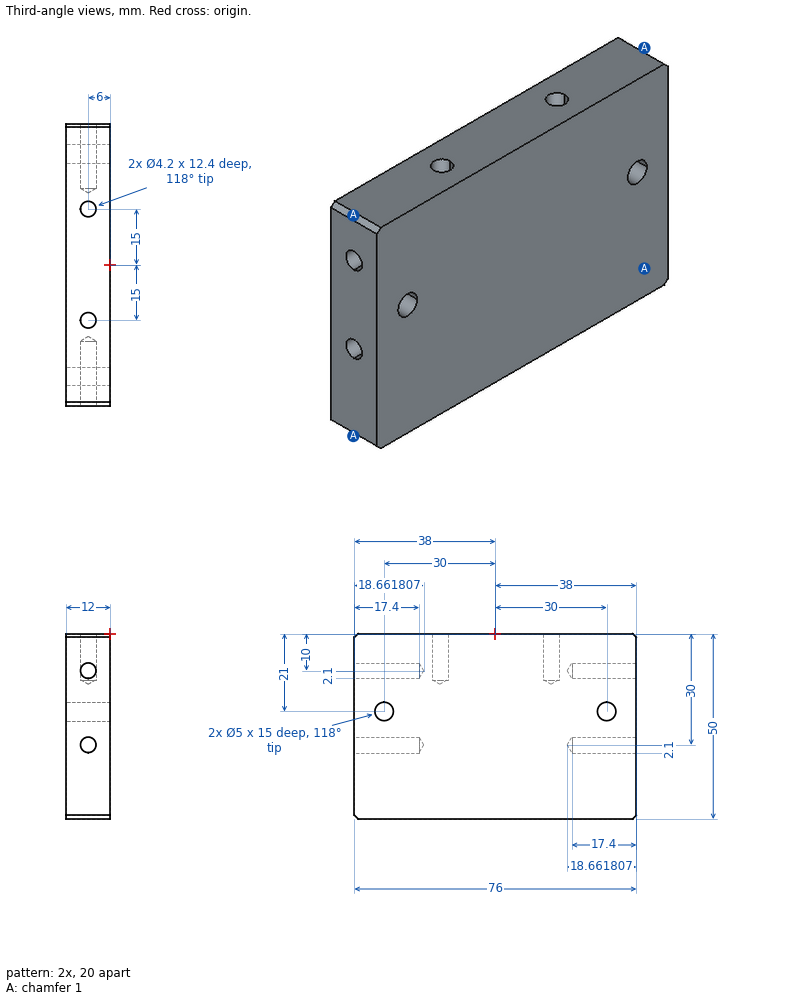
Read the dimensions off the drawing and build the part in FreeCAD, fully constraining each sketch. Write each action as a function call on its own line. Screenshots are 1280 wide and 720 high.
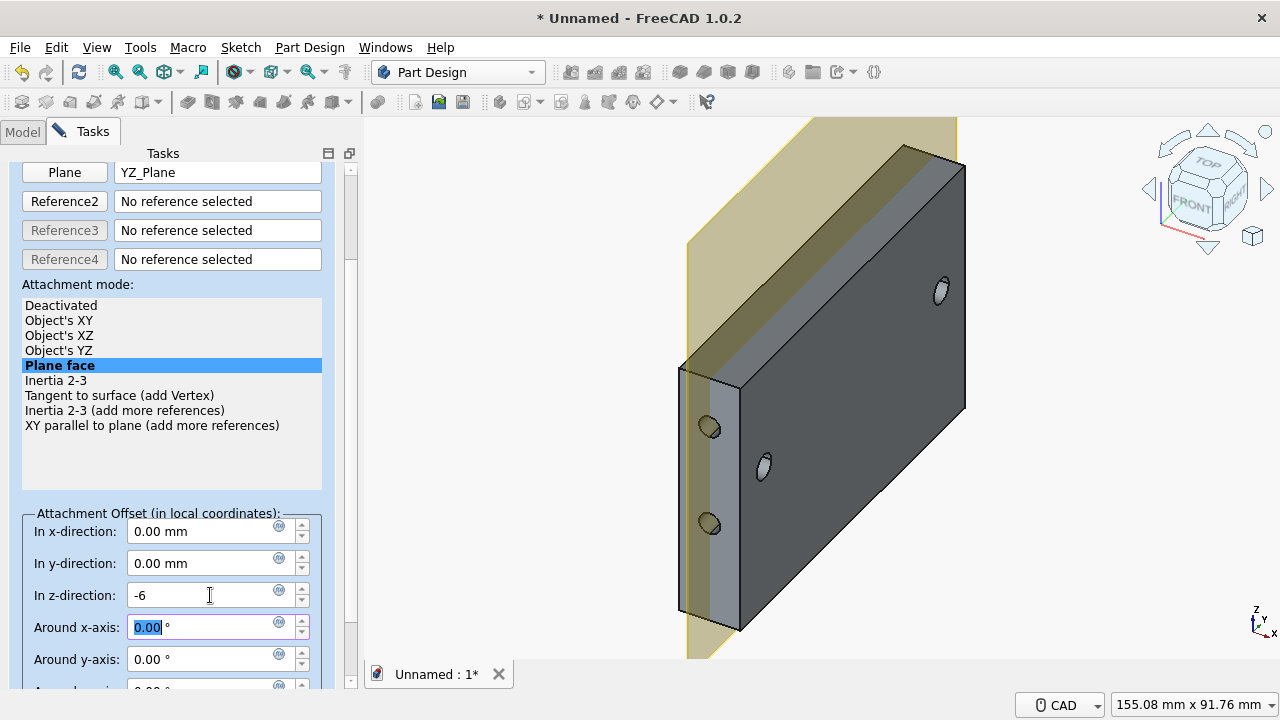
scroll(351, 426, up, 3)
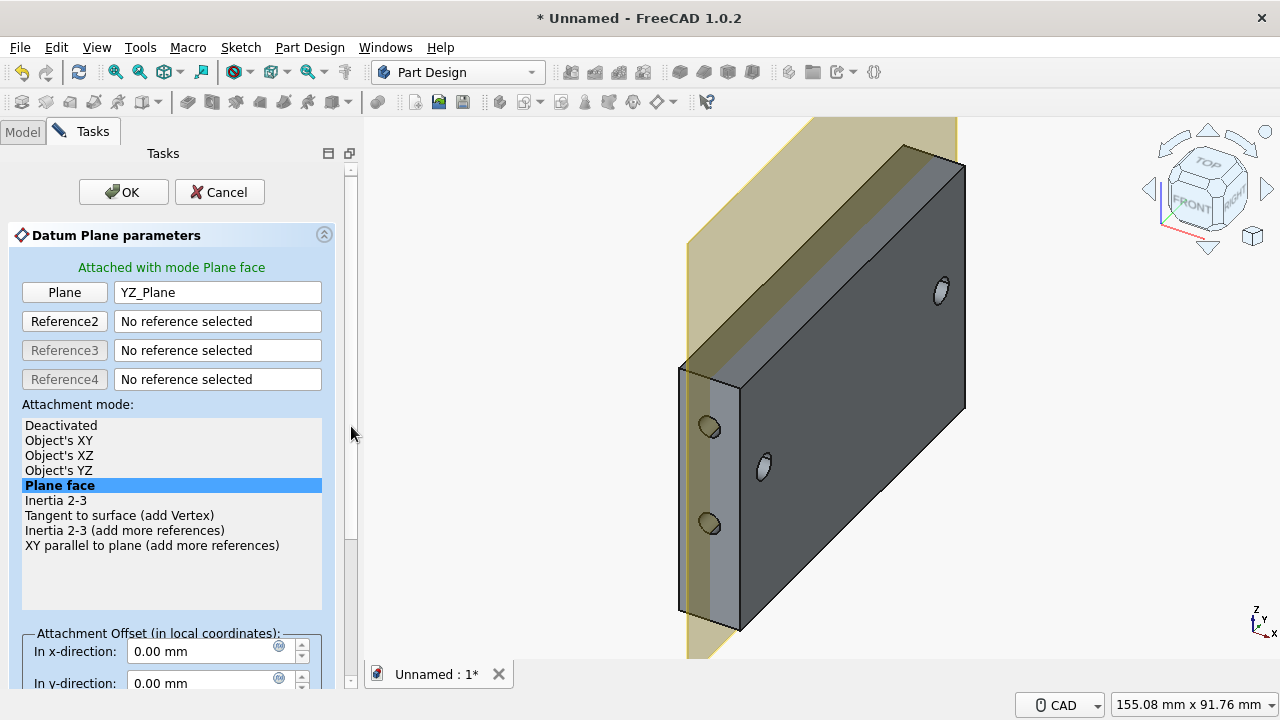
click(124, 192)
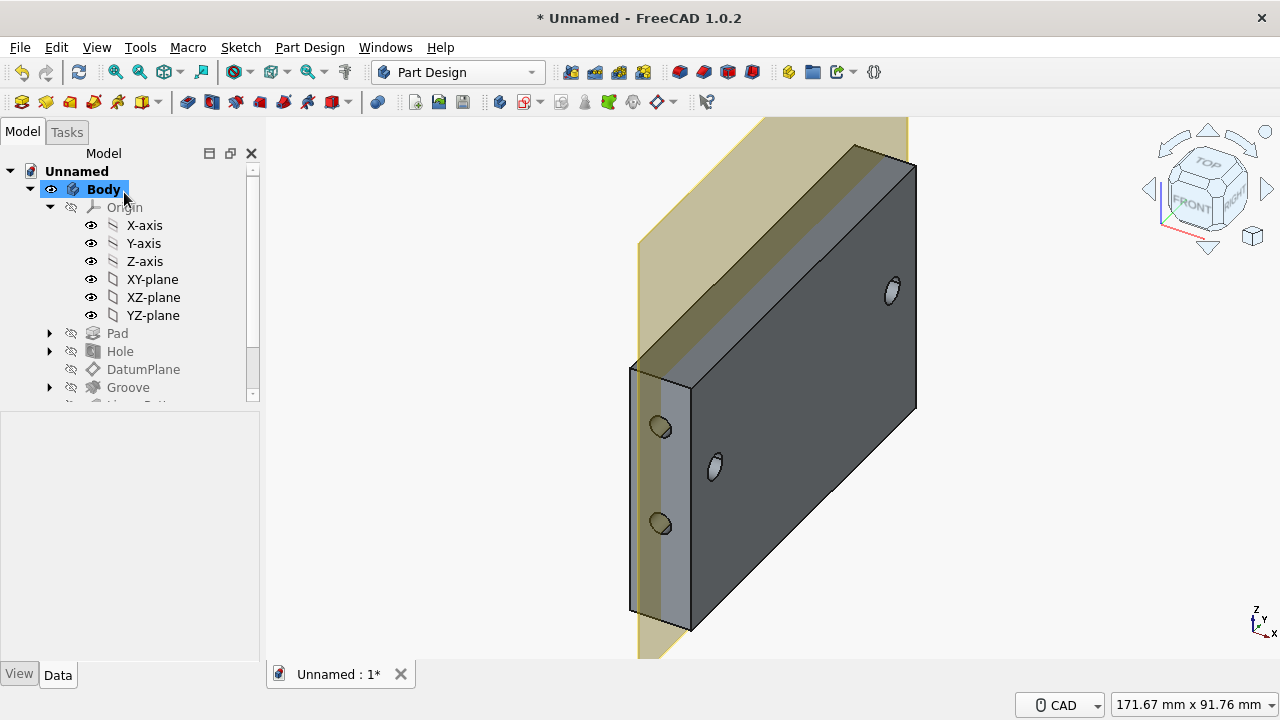
scroll(100, 275, down, 3)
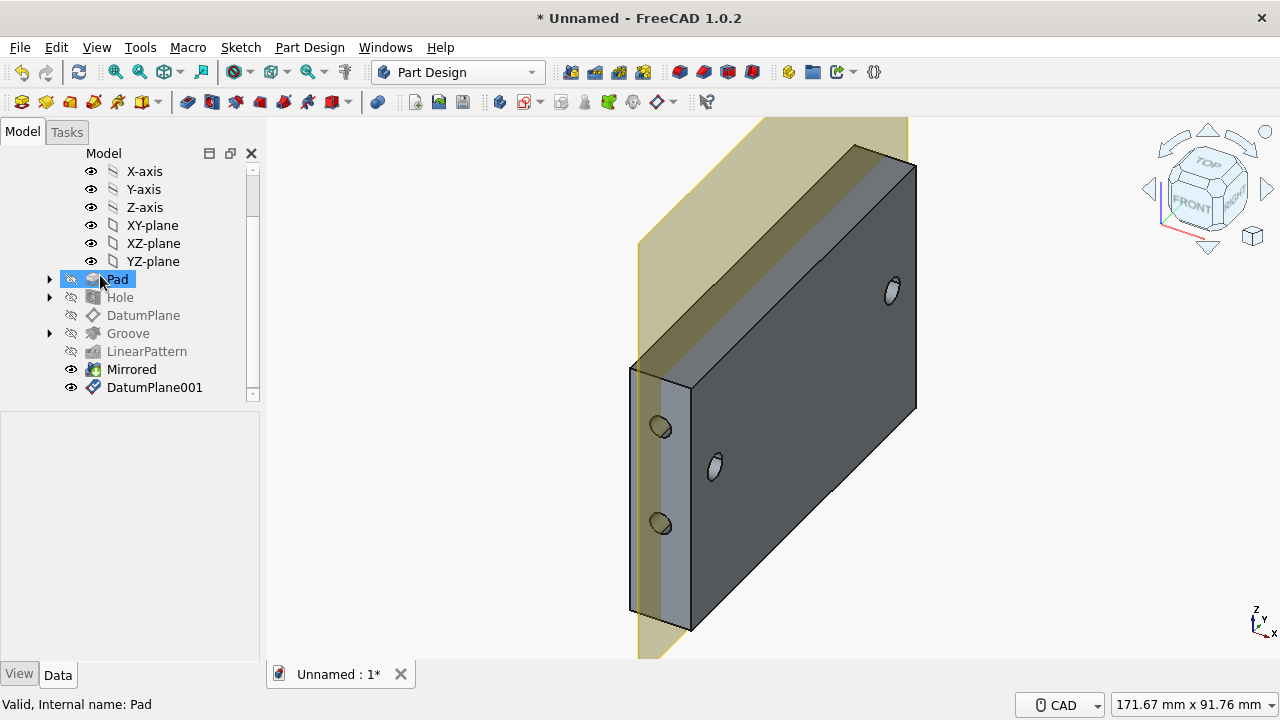
click(116, 387)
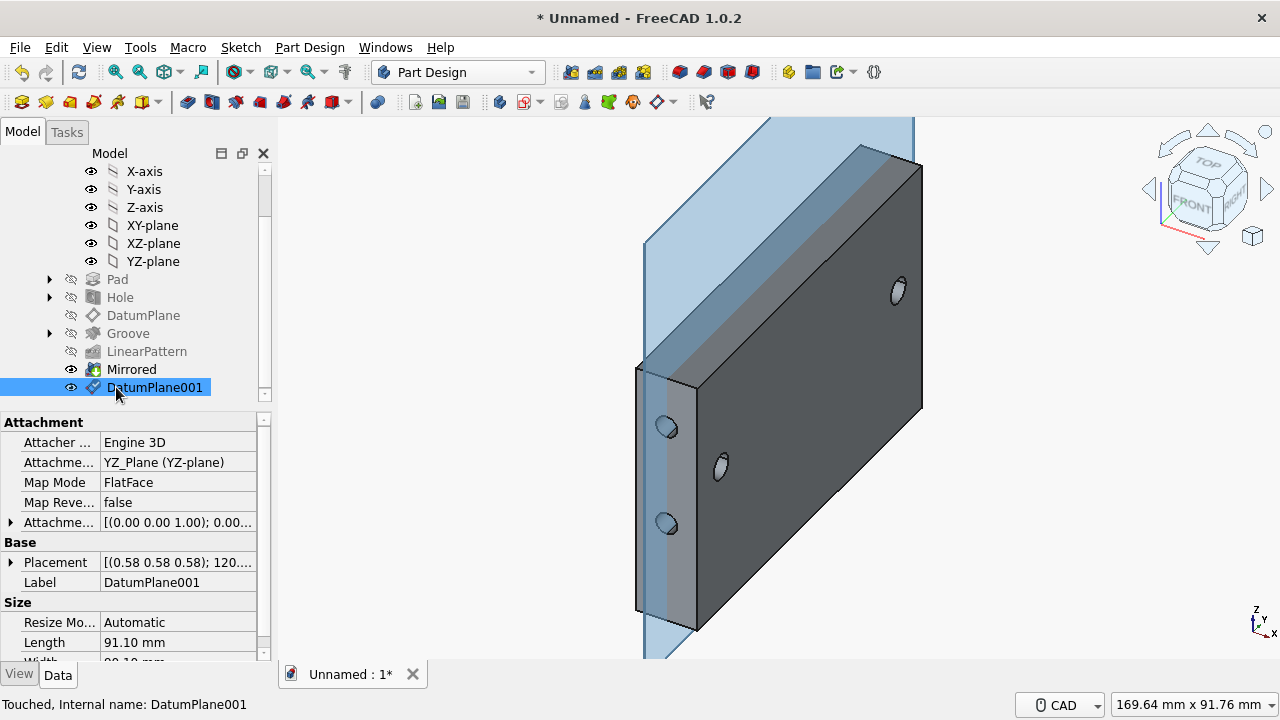
click(524, 102)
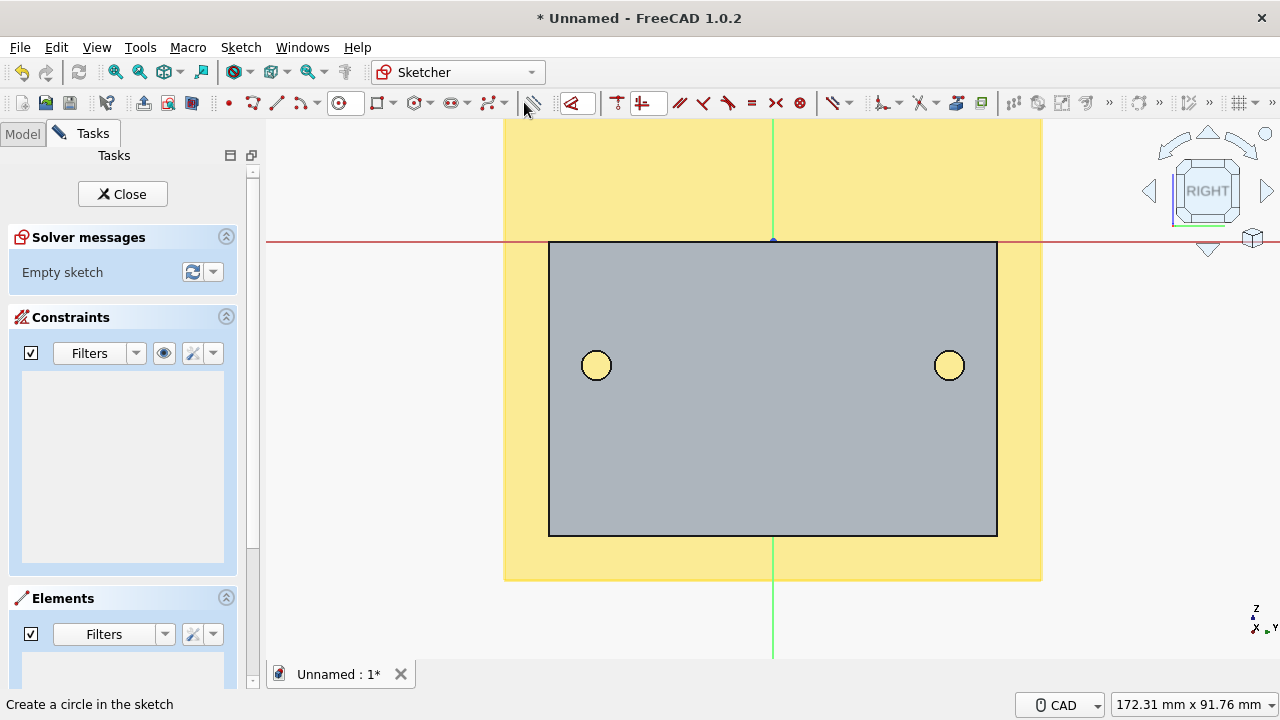
click(192, 104)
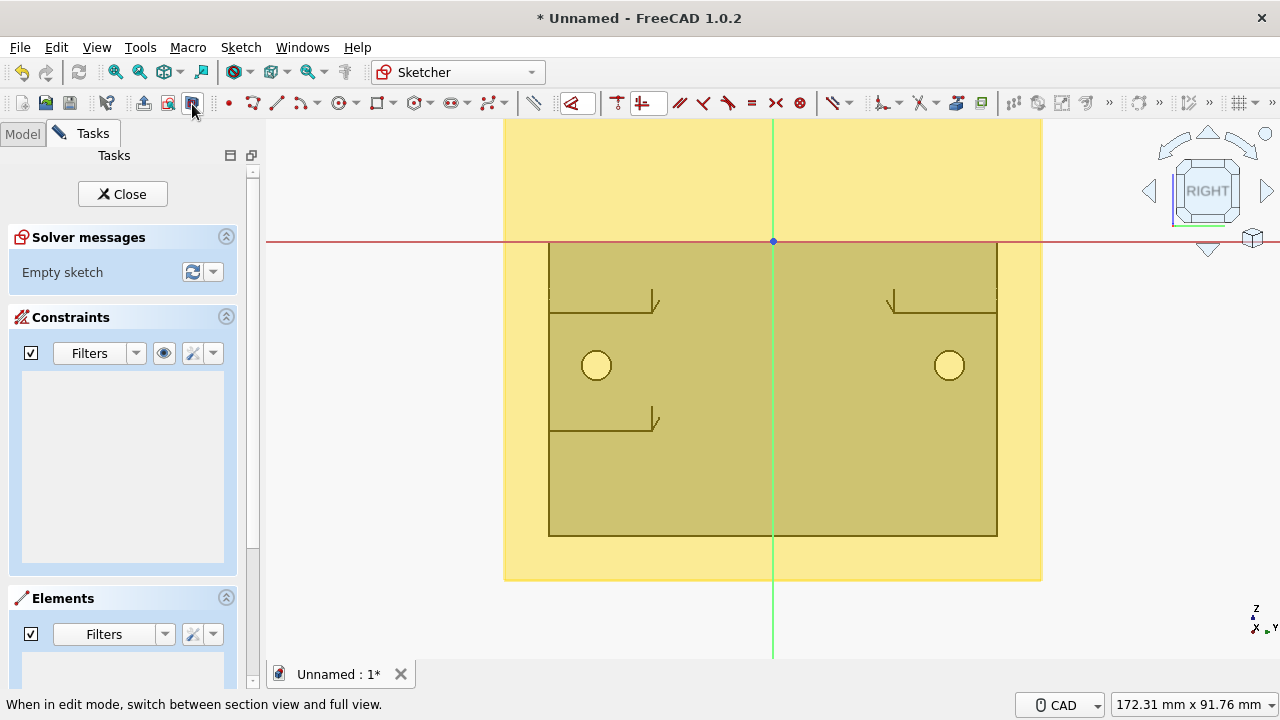
scroll(1115, 272, up, 3)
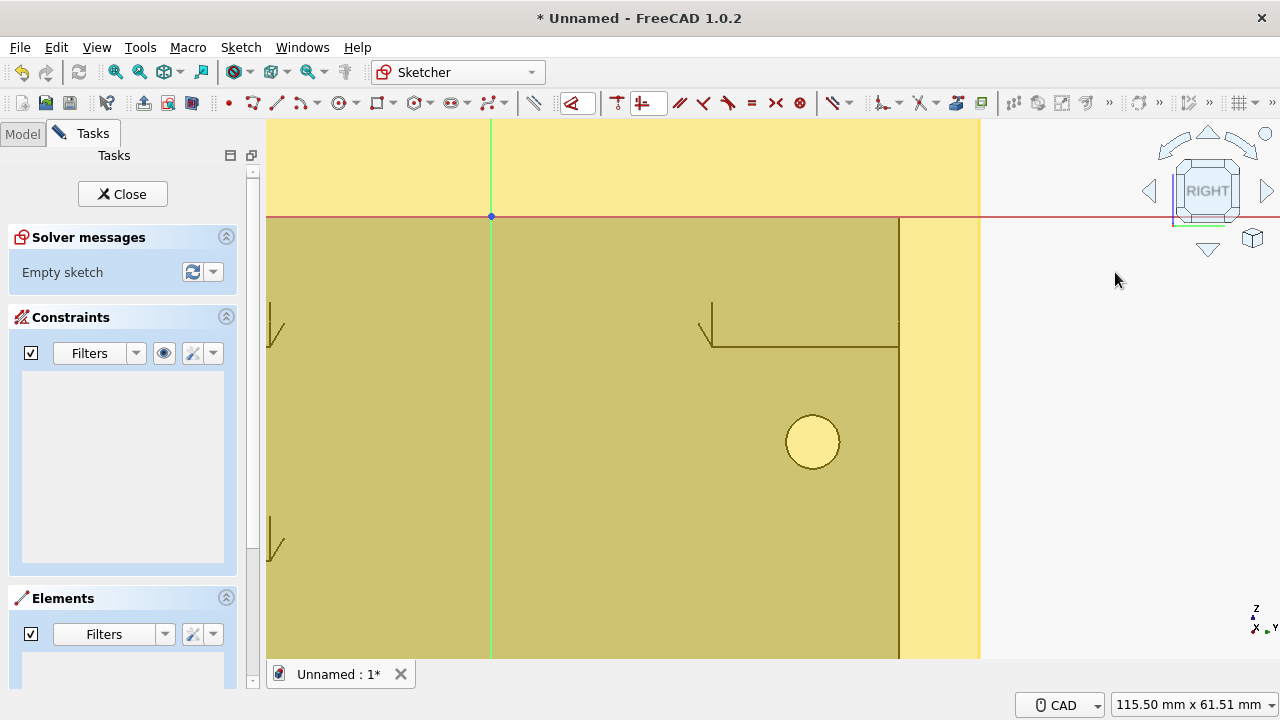
click(254, 104)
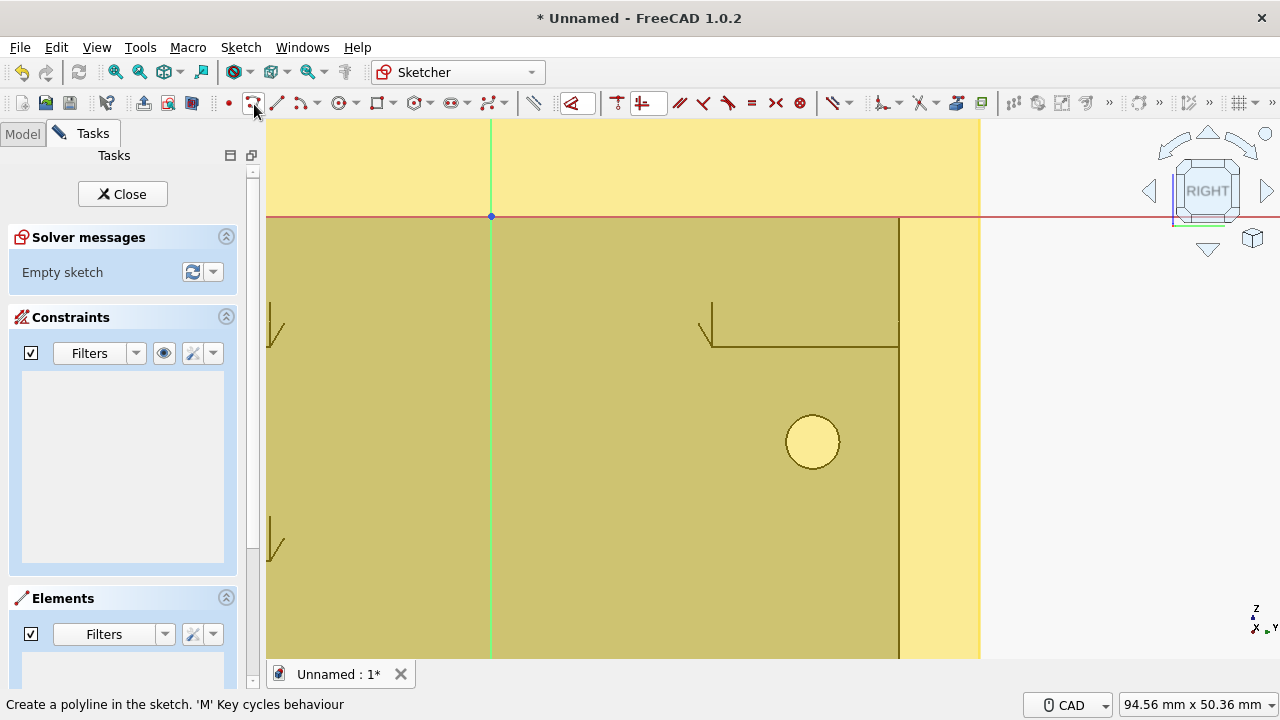
click(699, 539)
click(712, 561)
click(899, 561)
click(899, 539)
click(699, 540)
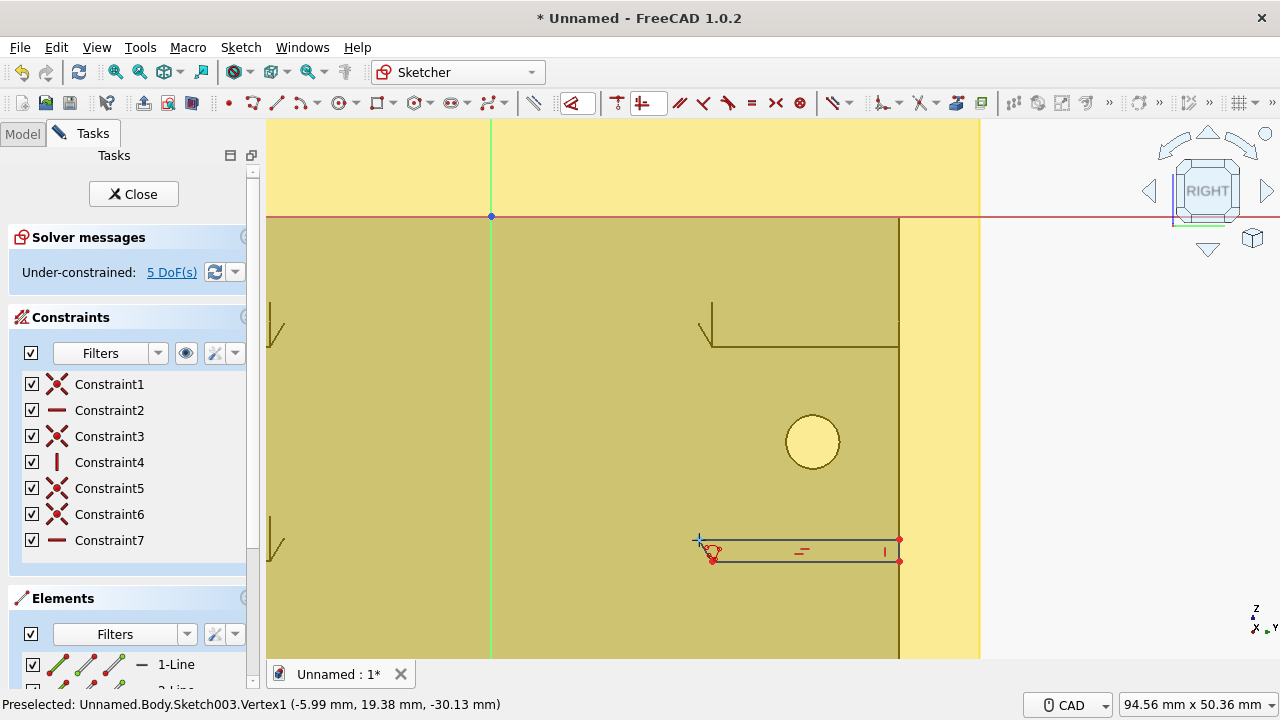
click(278, 104)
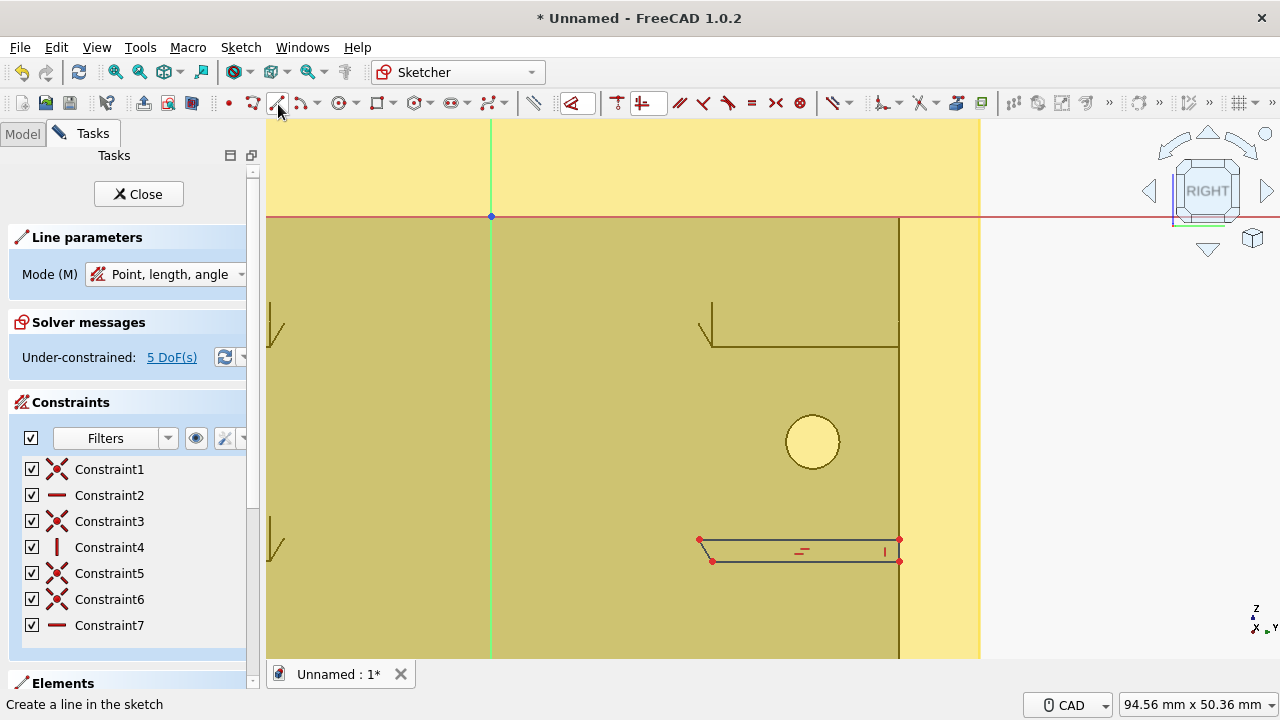
click(919, 539)
click(979, 539)
key(Escape)